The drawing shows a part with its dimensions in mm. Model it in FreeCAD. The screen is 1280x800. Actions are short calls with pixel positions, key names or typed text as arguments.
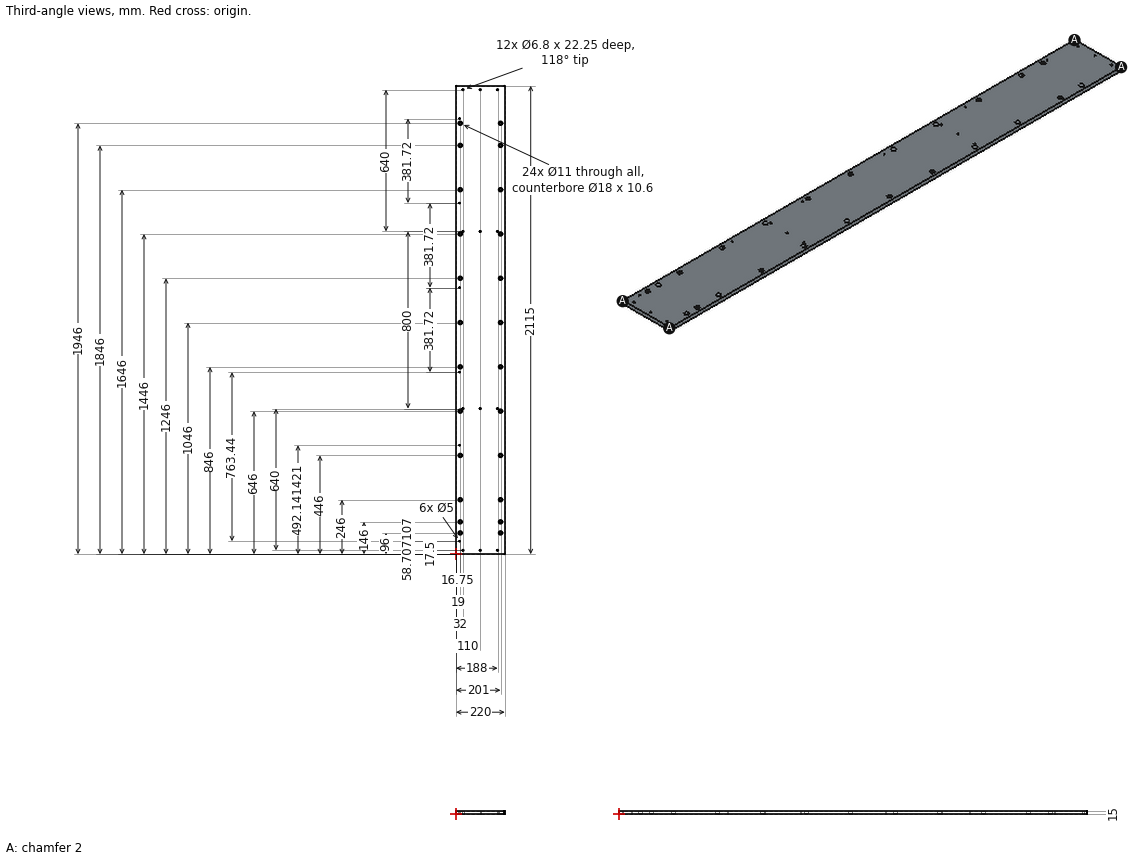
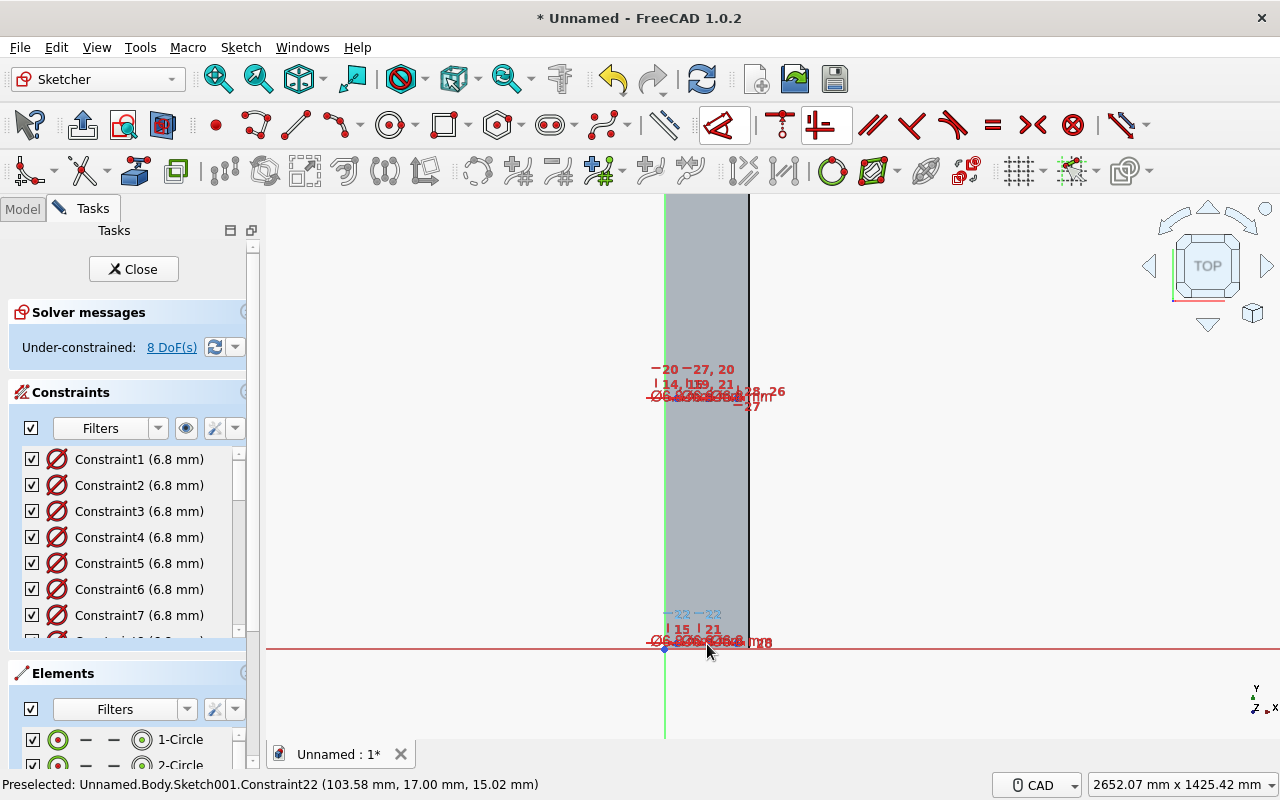
click(707, 643)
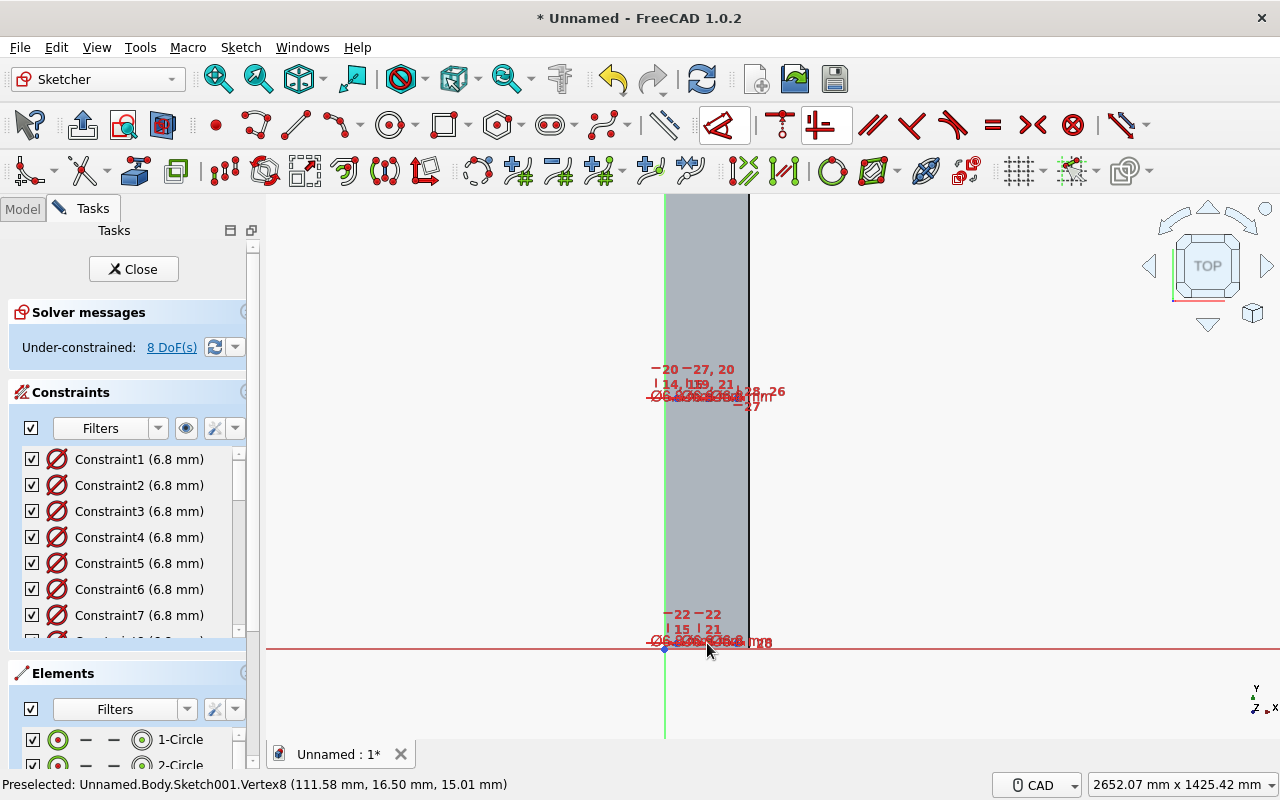
click(737, 643)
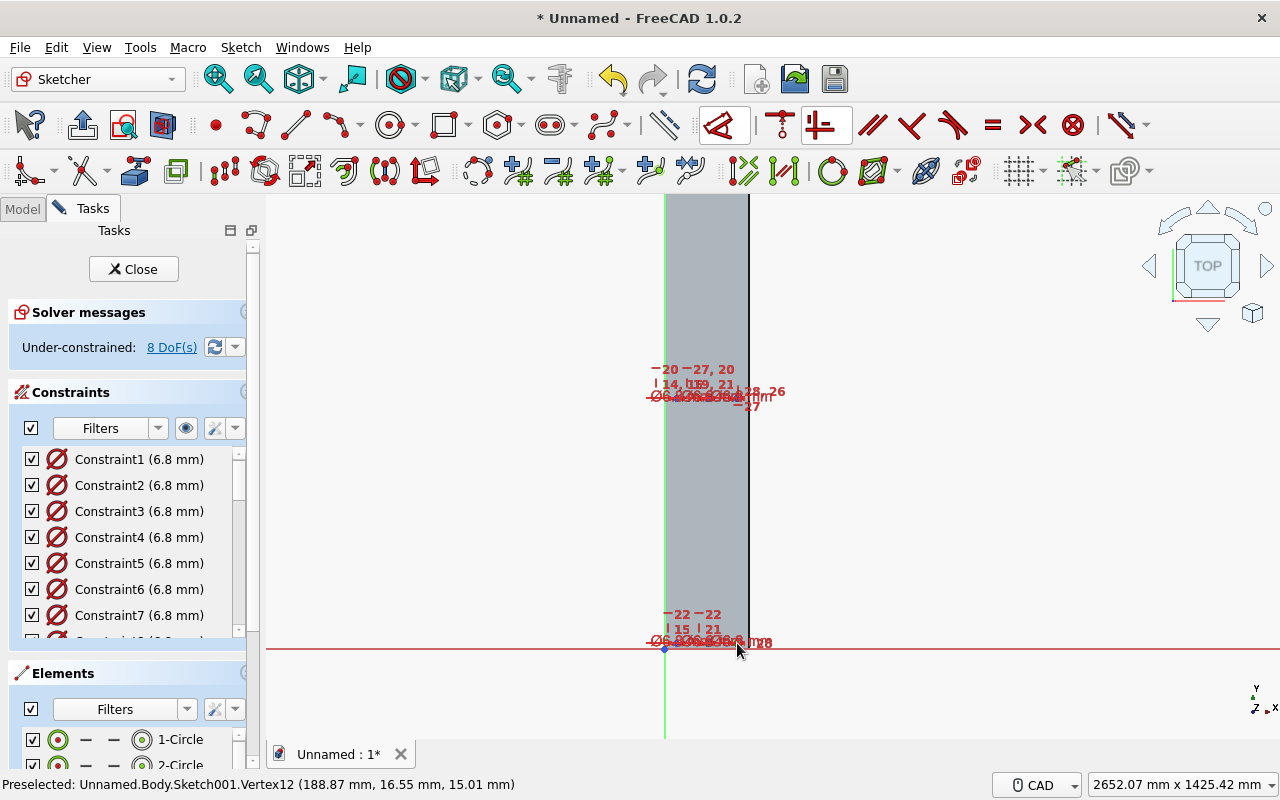
key(h)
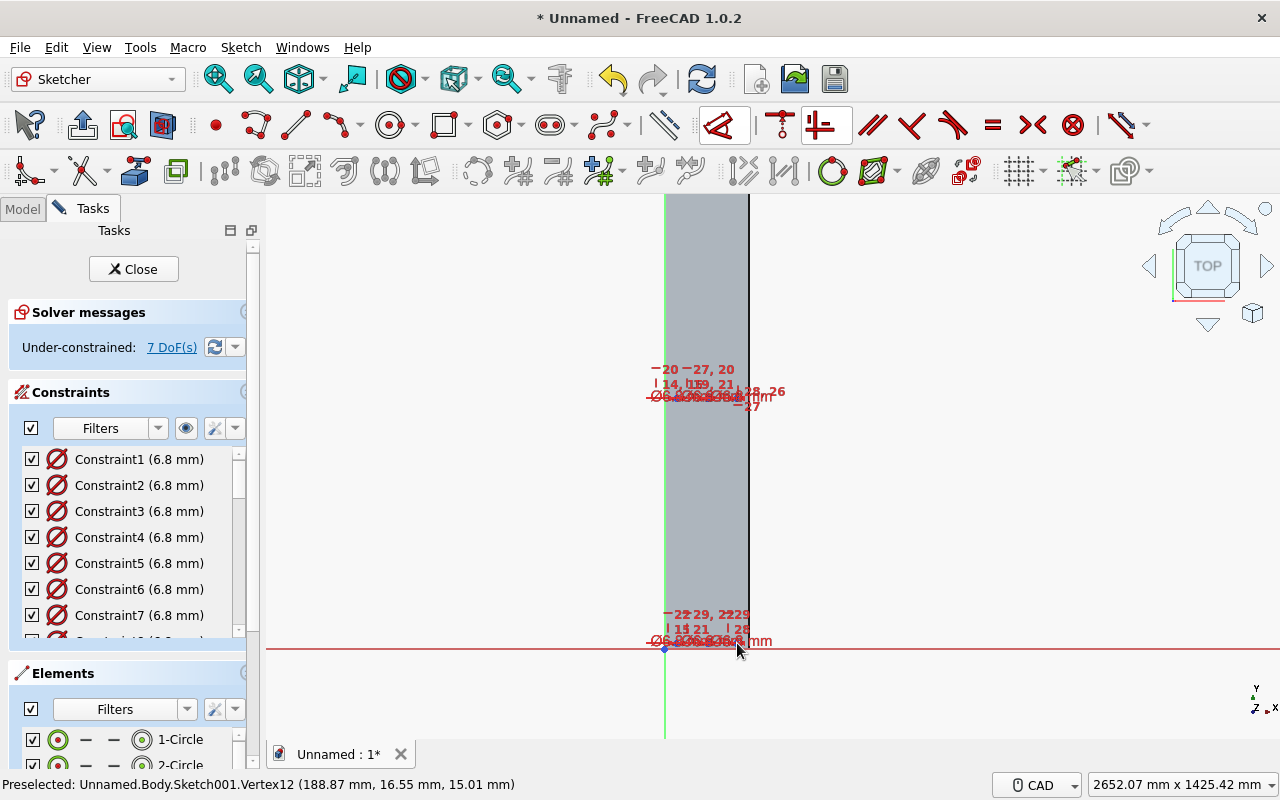
click(718, 126)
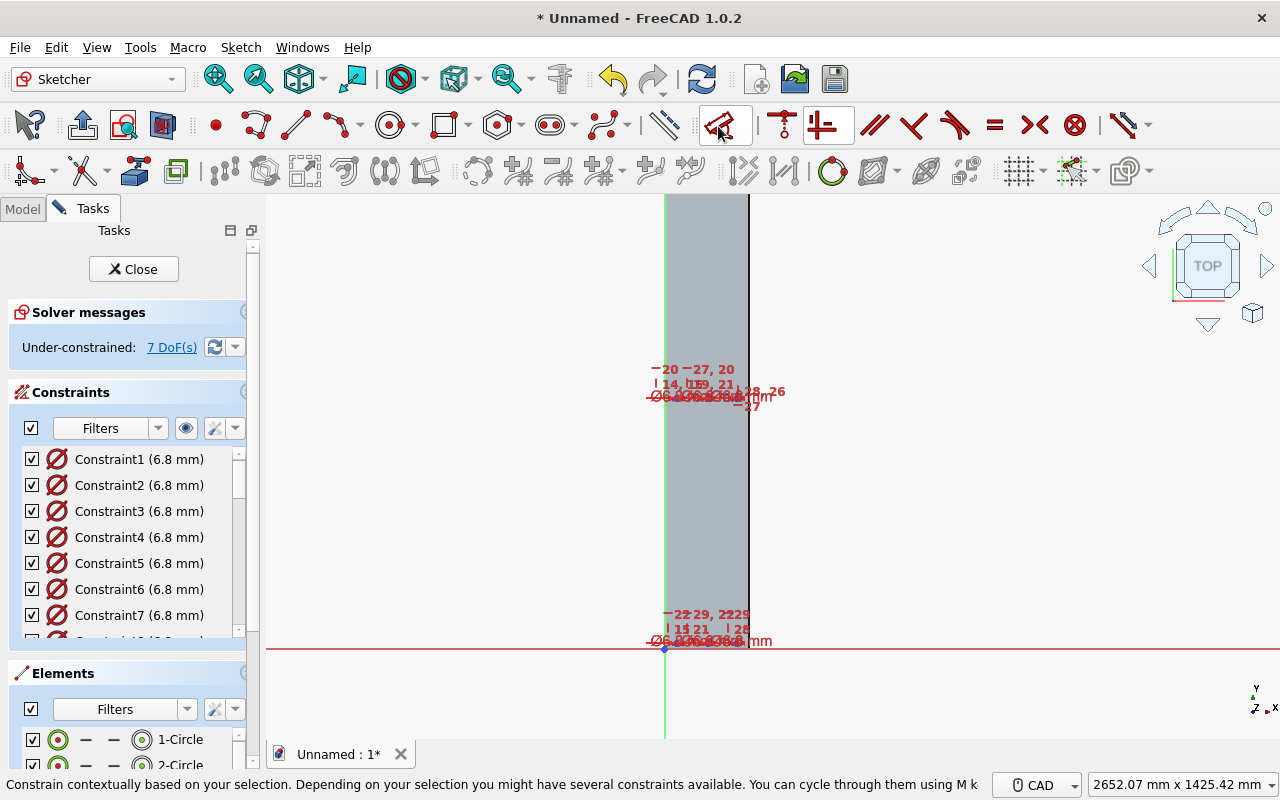
scroll(707, 645, down, 4)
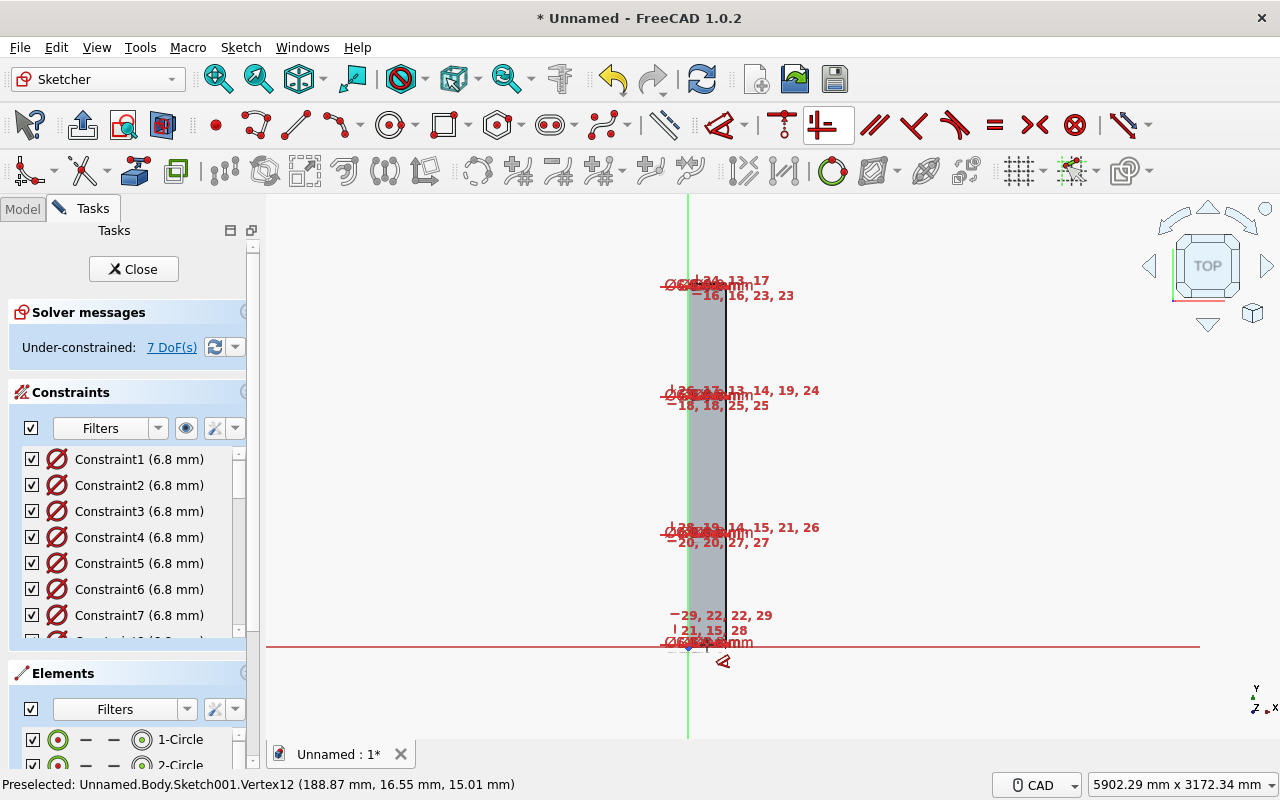
scroll(694, 287, up, 10)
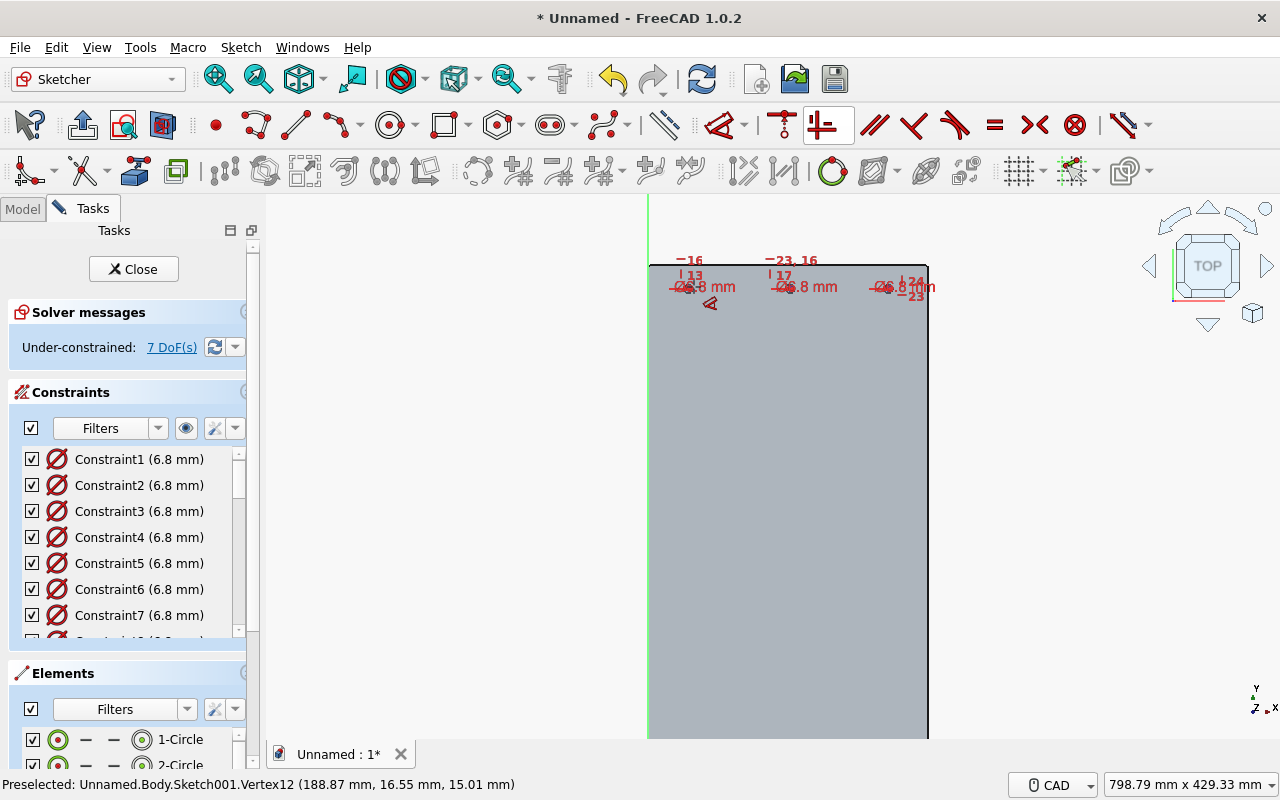
click(688, 289)
click(668, 255)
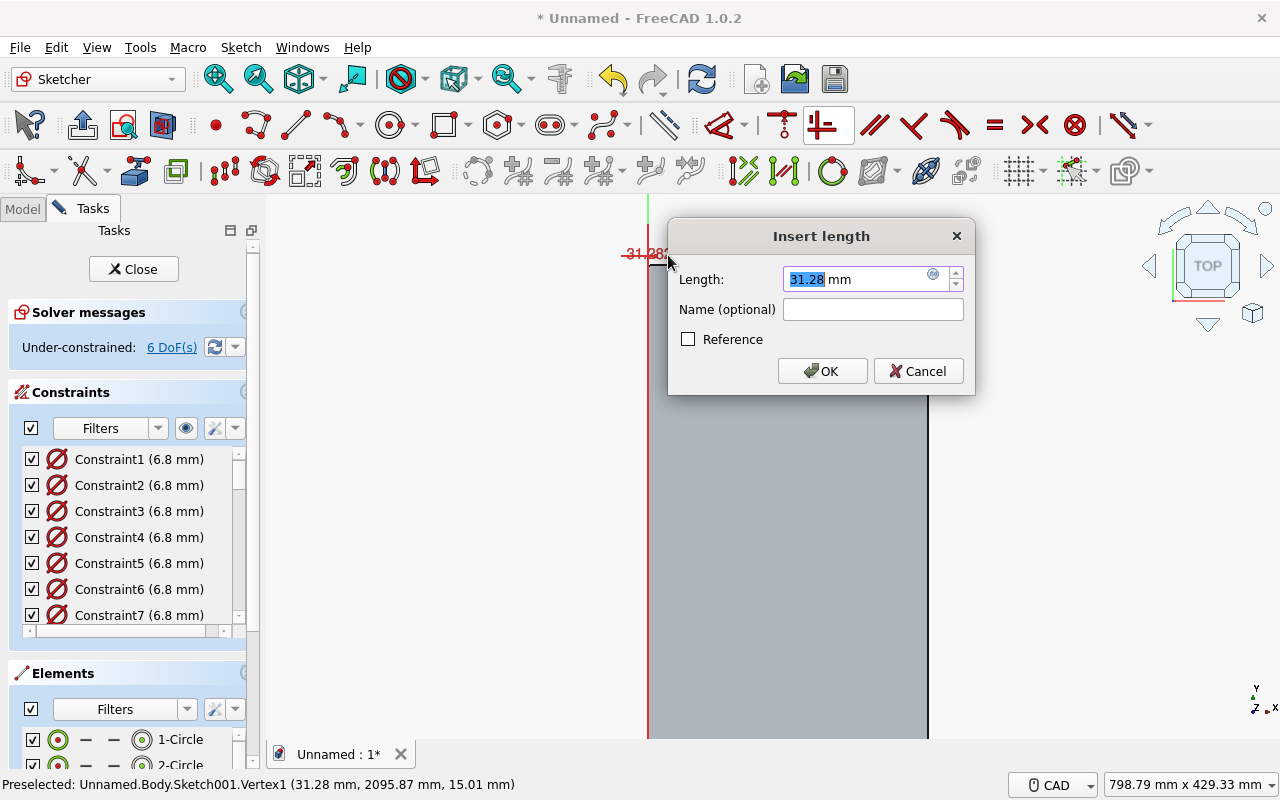
text(32)
key(Return)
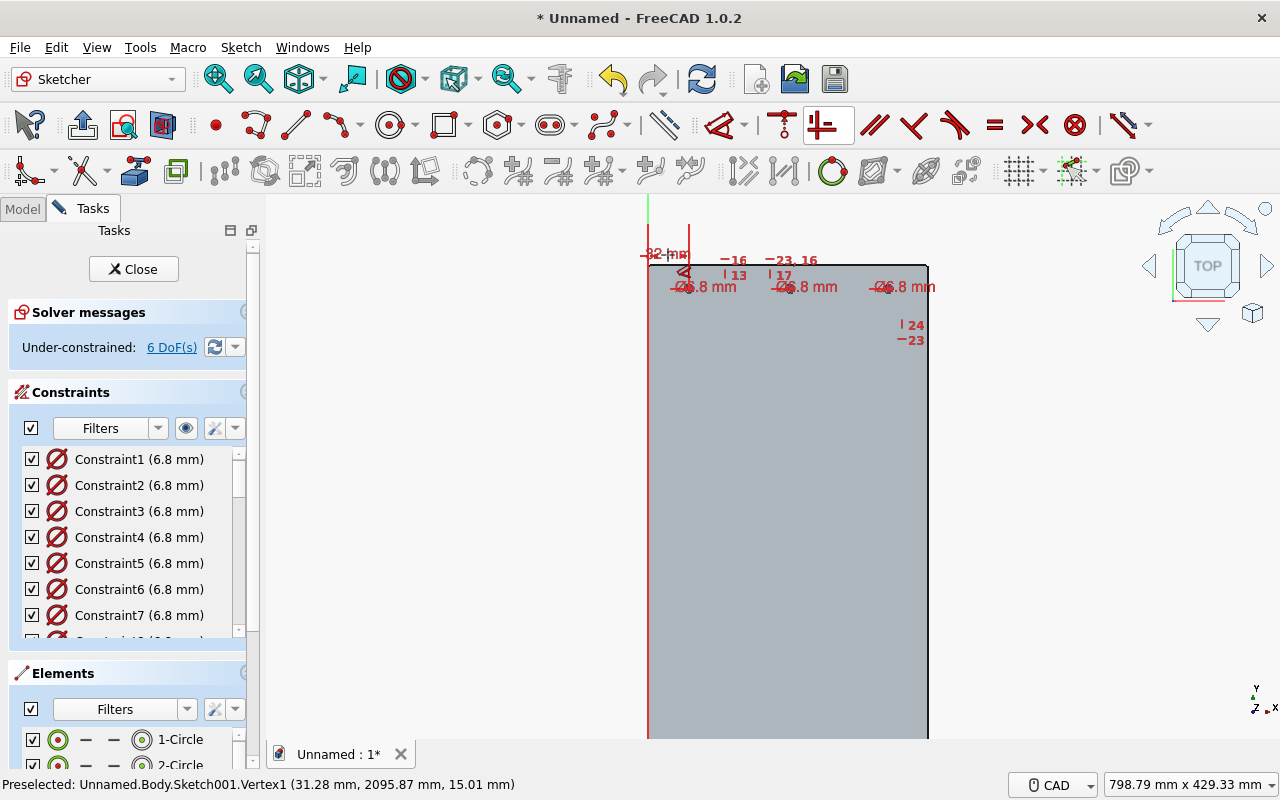
scroll(694, 287, down, 10)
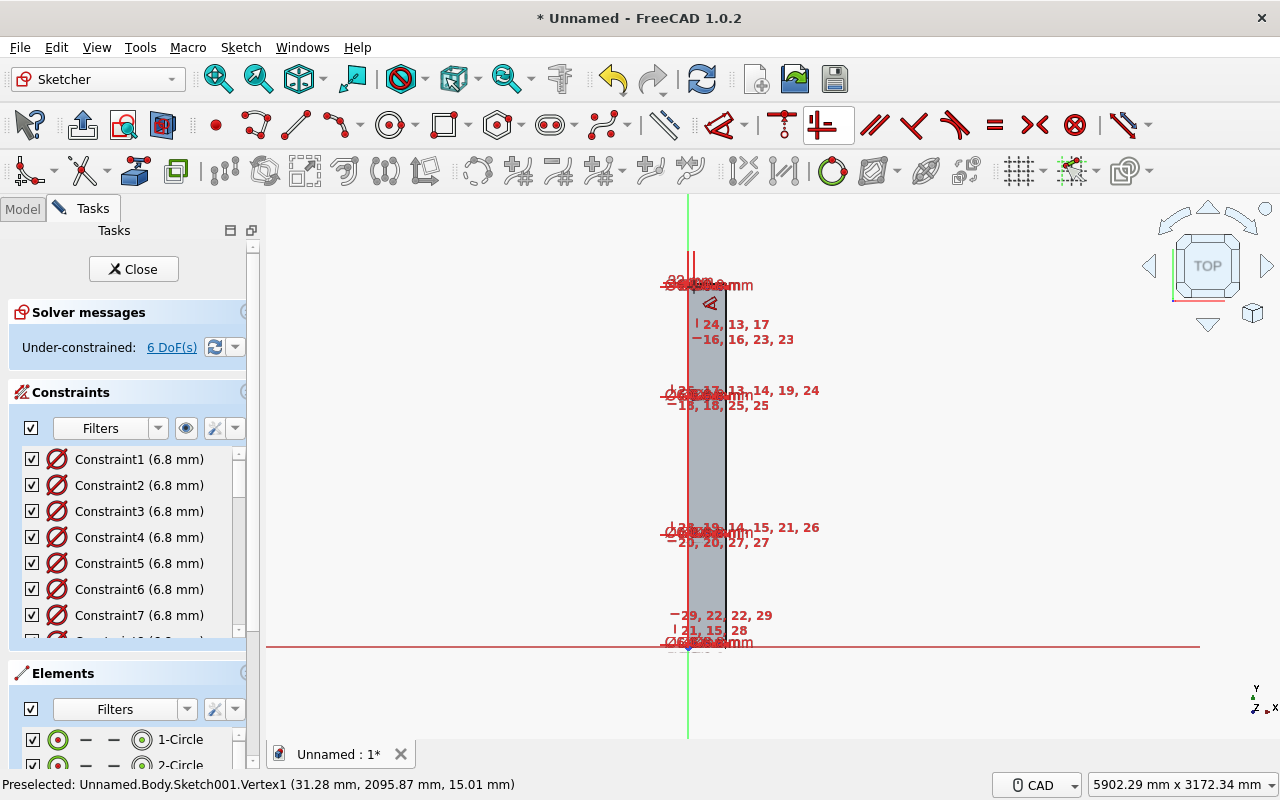
scroll(707, 287, up, 4)